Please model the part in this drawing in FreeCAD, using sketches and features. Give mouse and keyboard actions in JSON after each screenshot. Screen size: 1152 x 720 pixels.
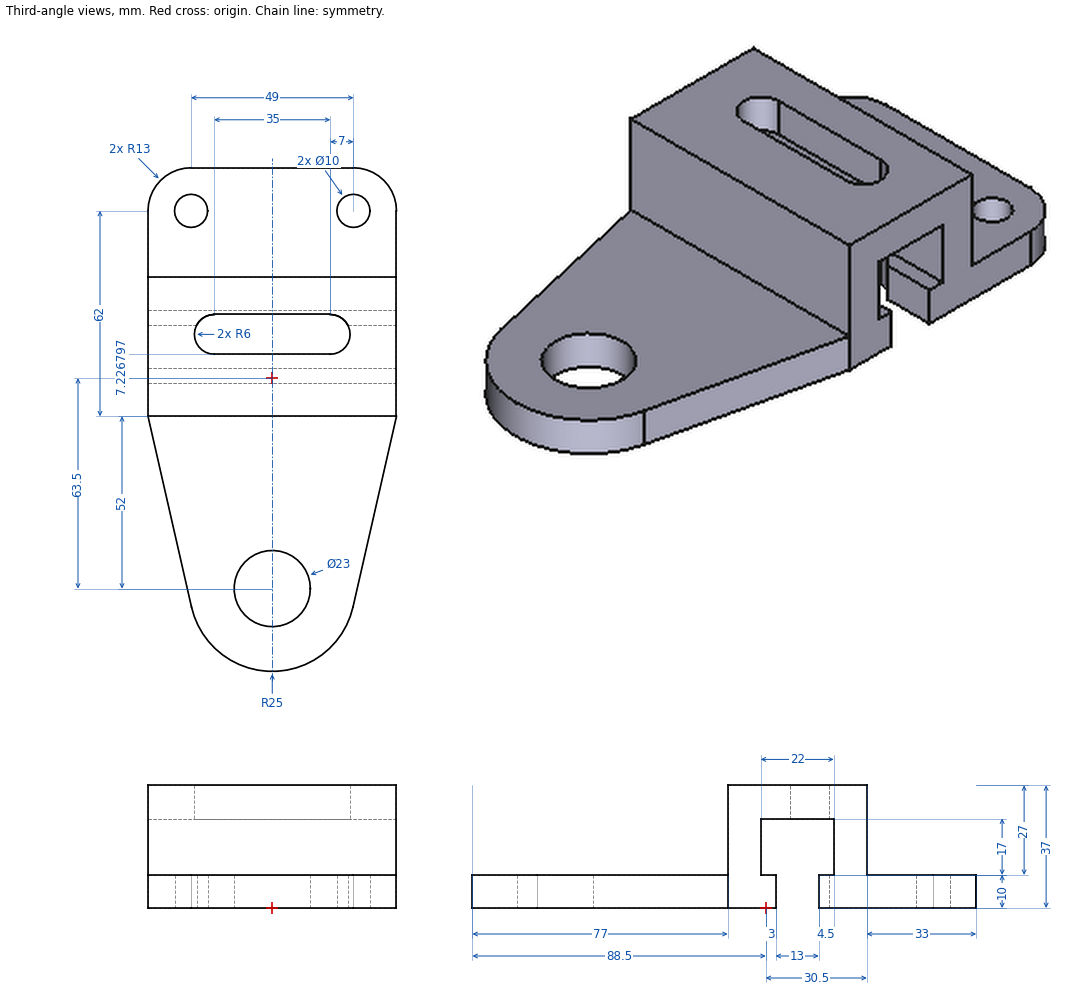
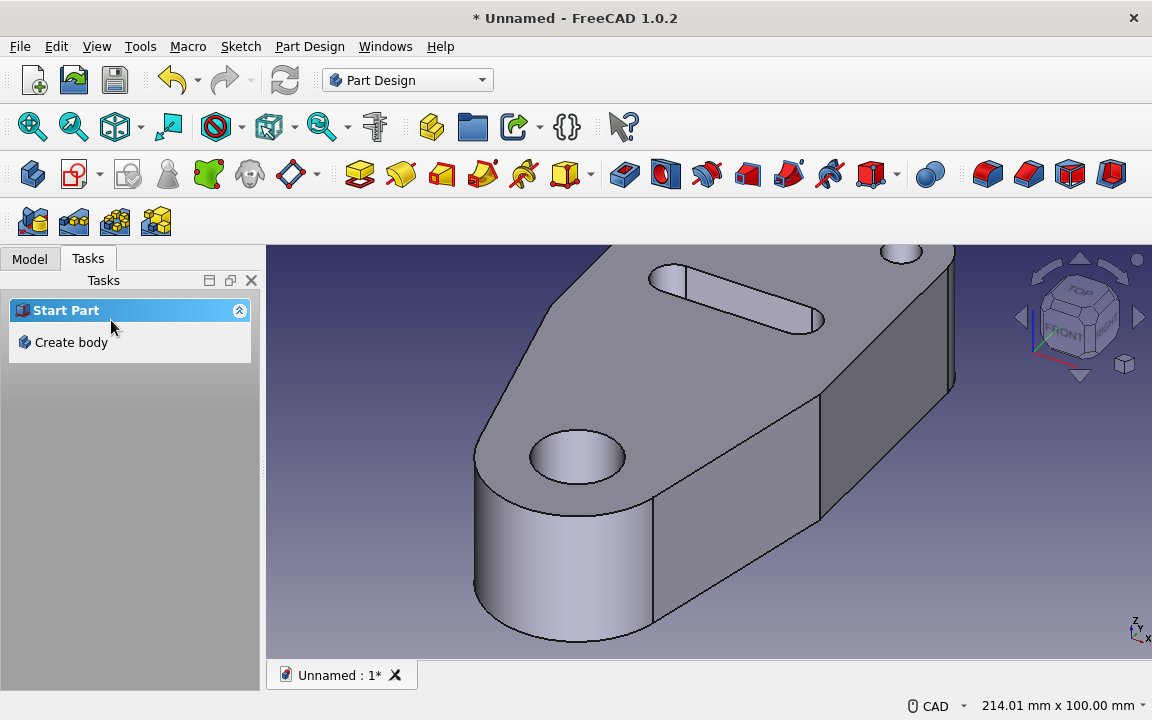
{"action": "left_click", "coordinate": [33, 128]}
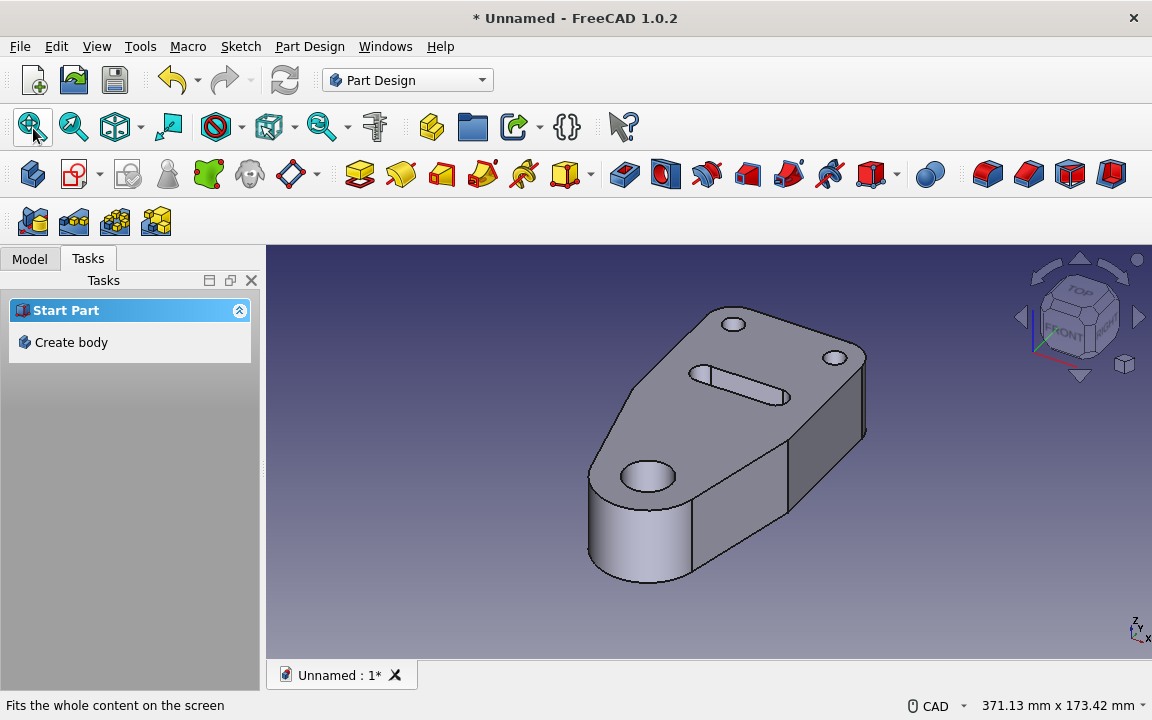
{"action": "left_click", "coordinate": [74, 174]}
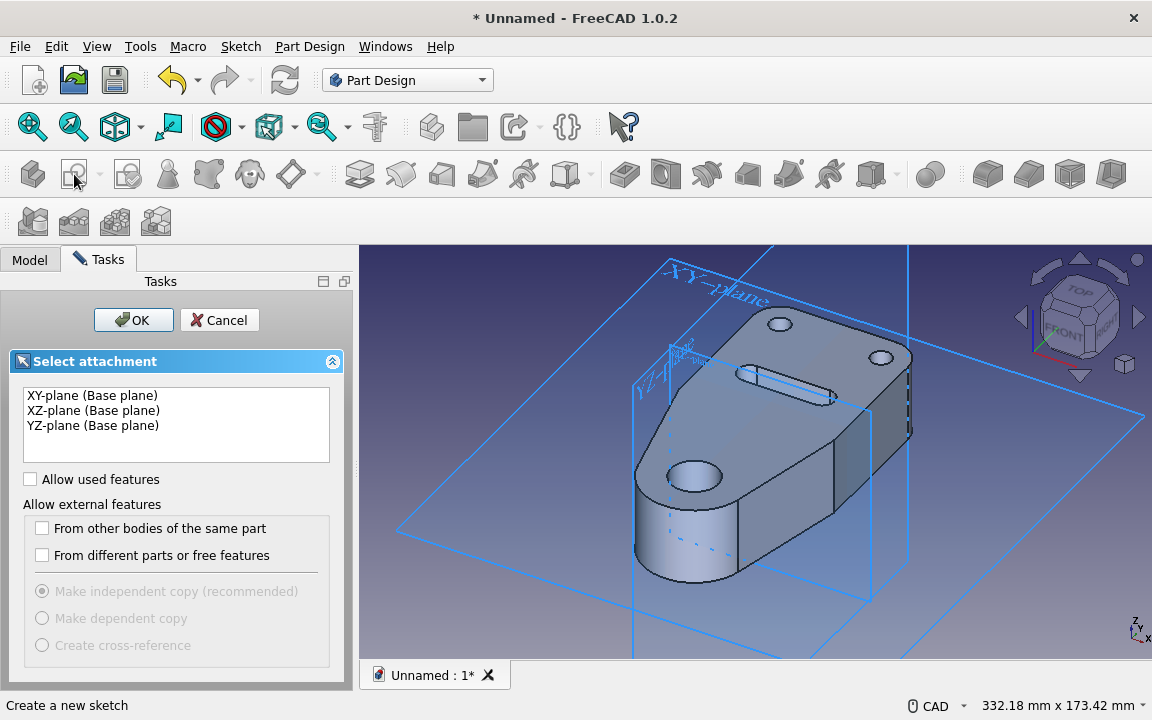
{"action": "left_click", "coordinate": [84, 426]}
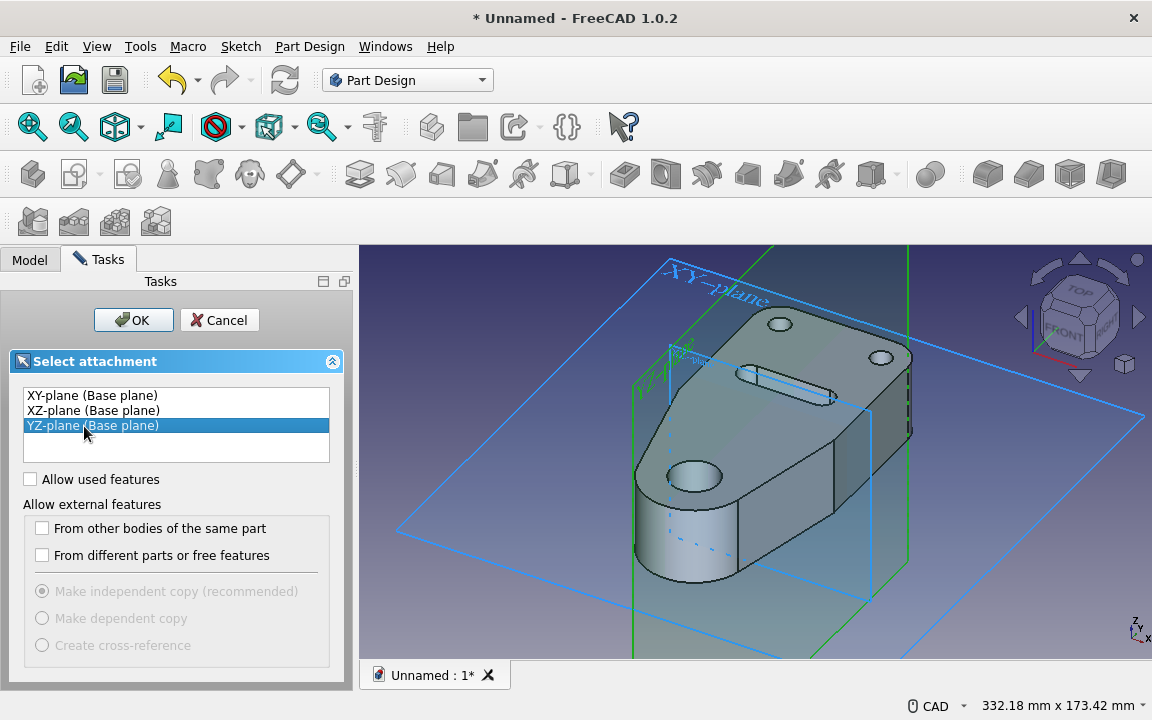
{"action": "left_click", "coordinate": [134, 320]}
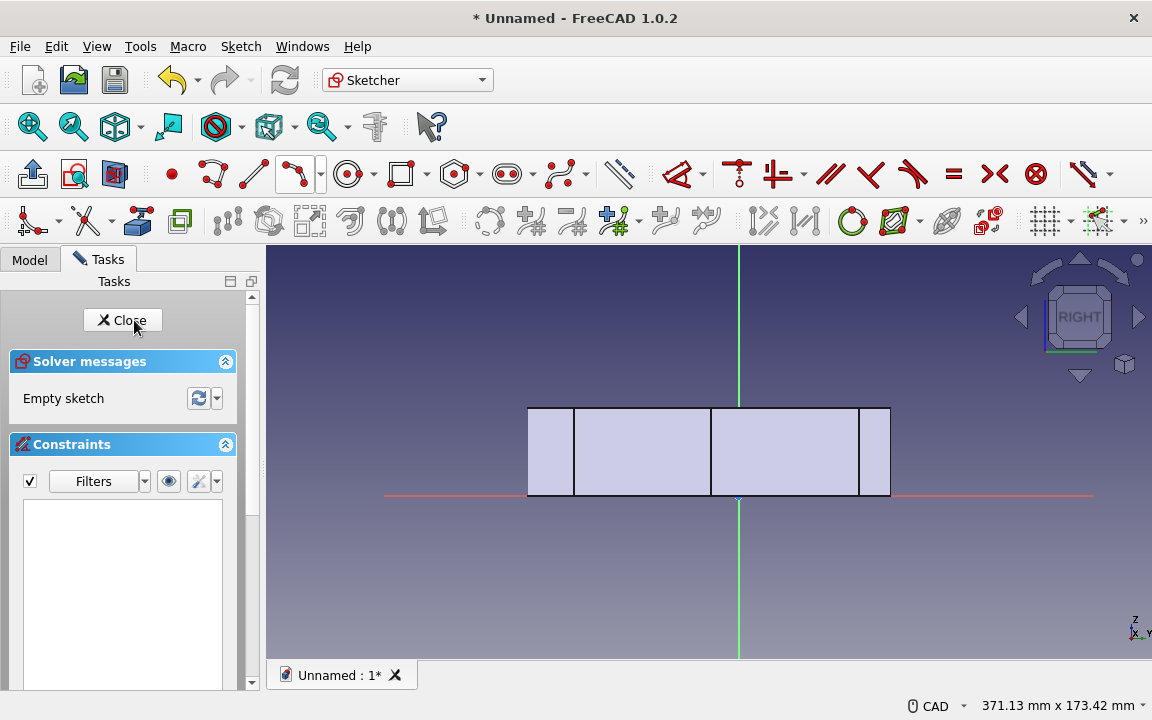
{"action": "left_click", "coordinate": [115, 174]}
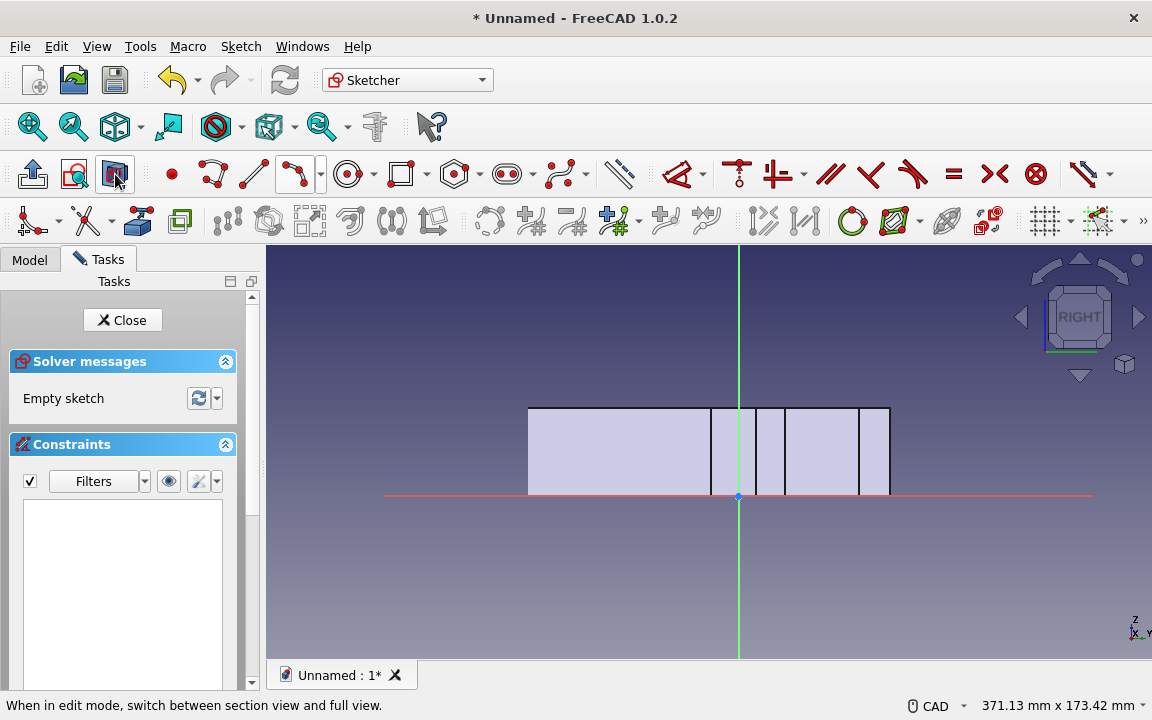
{"action": "left_click", "coordinate": [400, 174]}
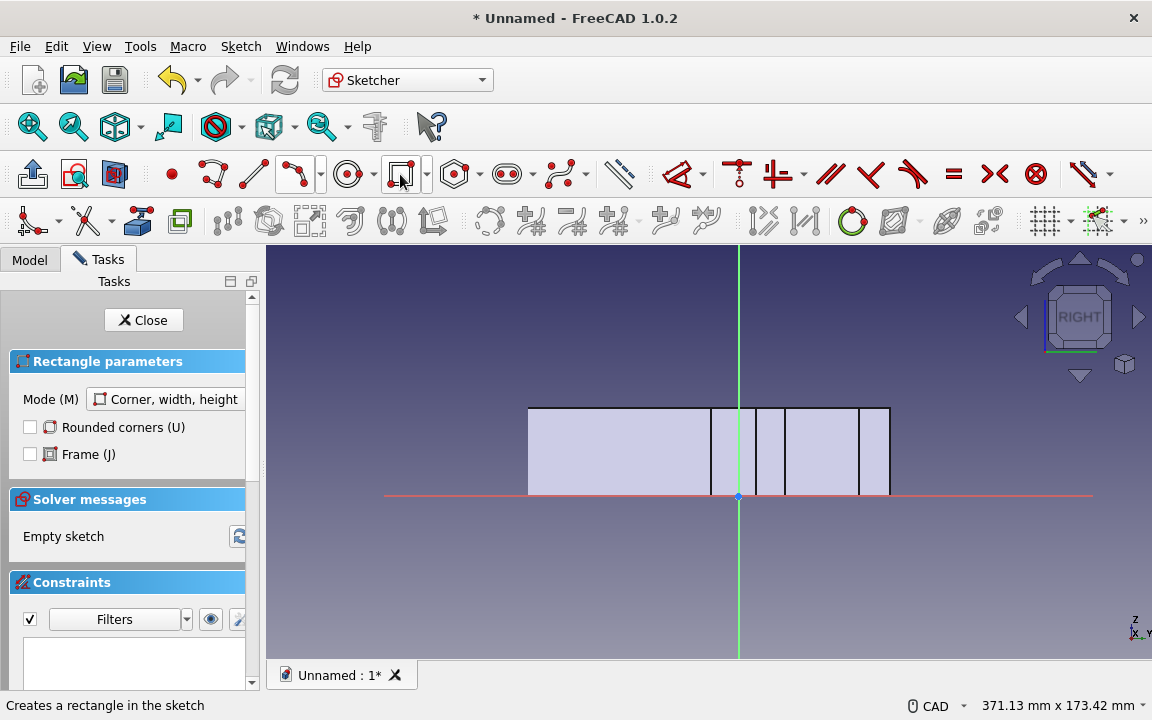
{"action": "left_click", "coordinate": [812, 408]}
{"action": "mouse_move", "coordinate": [890, 472]}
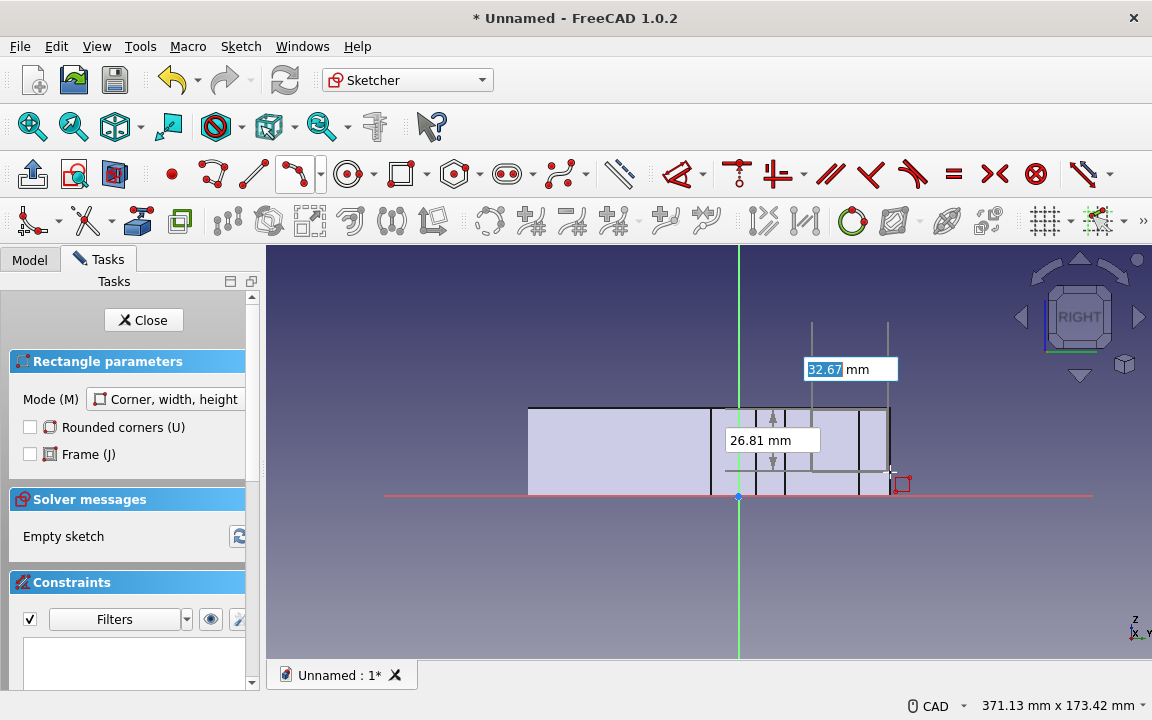
{"action": "type", "text": "33"}
{"action": "key", "text": "Tab"}
{"action": "type", "text": "27"}
{"action": "key", "text": "Return"}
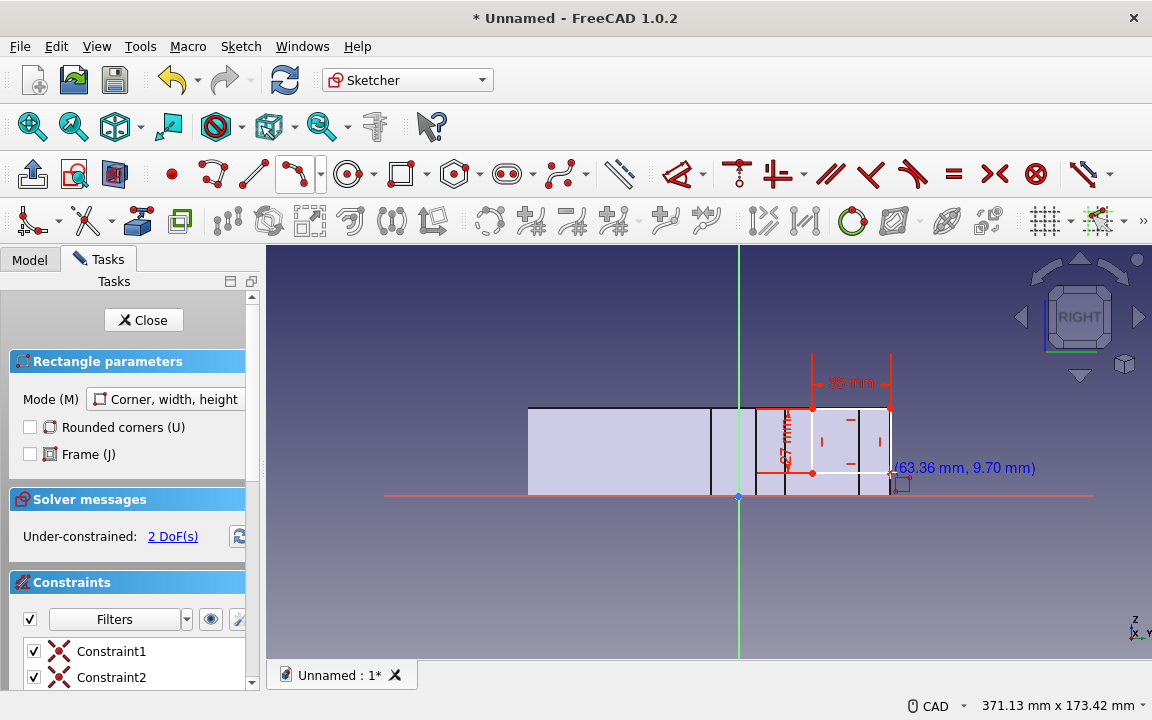
{"action": "left_click", "coordinate": [213, 174]}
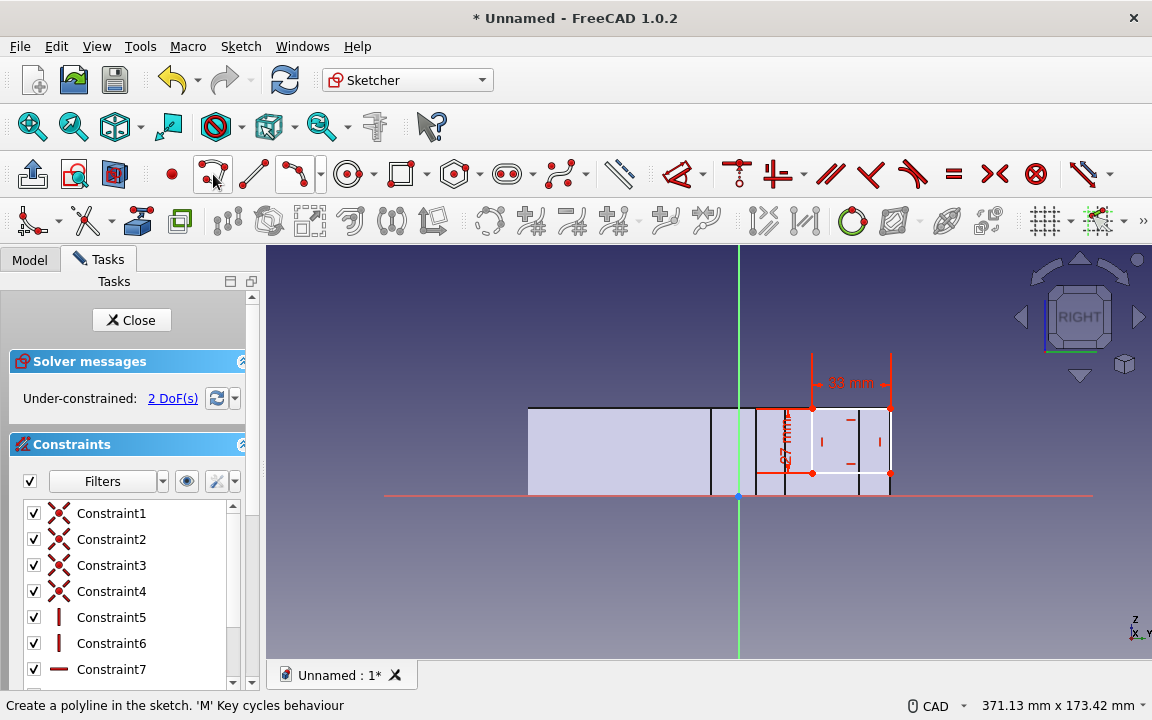
{"action": "scroll", "coordinate": [746, 496], "scroll_direction": "up", "scroll_amount": 4}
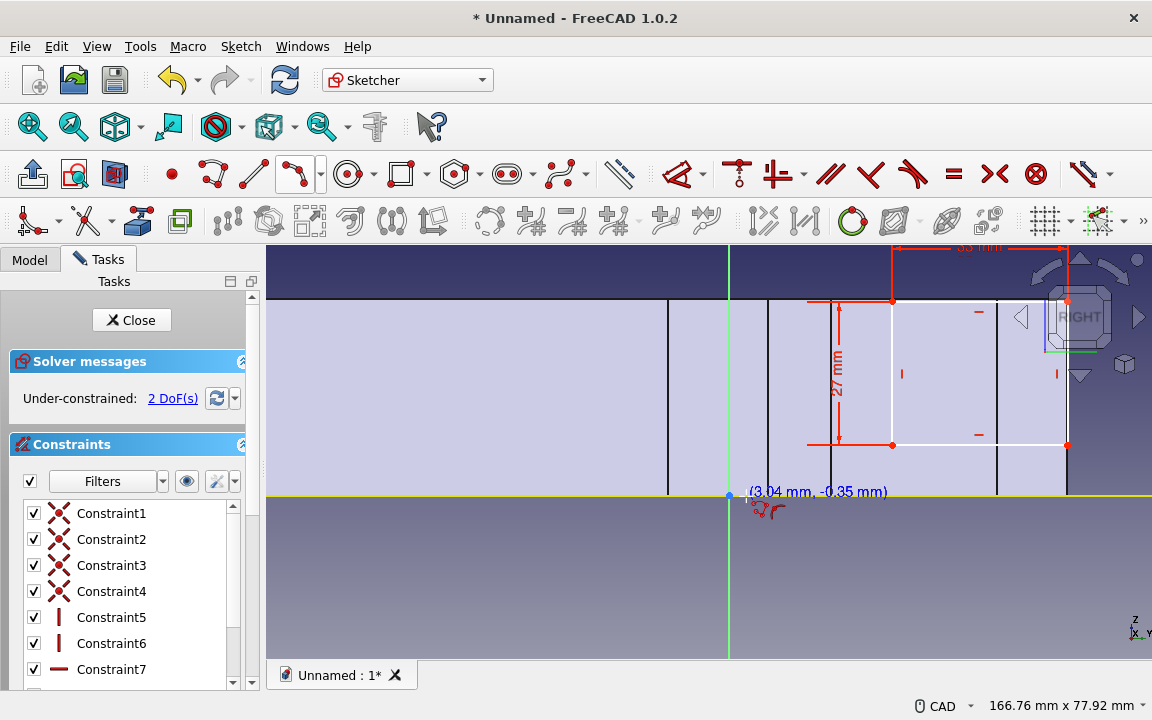
{"action": "left_click", "coordinate": [745, 496]}
{"action": "left_click", "coordinate": [814, 487]}
{"action": "left_click", "coordinate": [814, 442]}
{"action": "left_click", "coordinate": [838, 442]}
{"action": "left_click", "coordinate": [838, 352]}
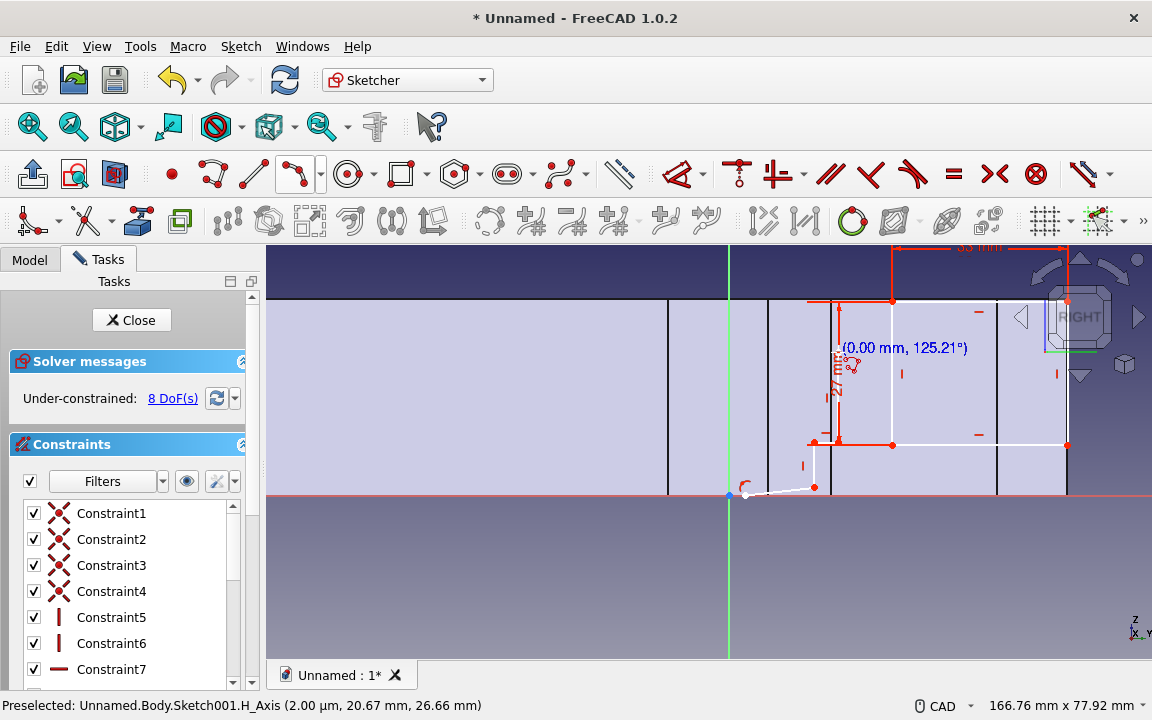
{"action": "scroll", "coordinate": [721, 352], "scroll_direction": "up", "scroll_amount": 4}